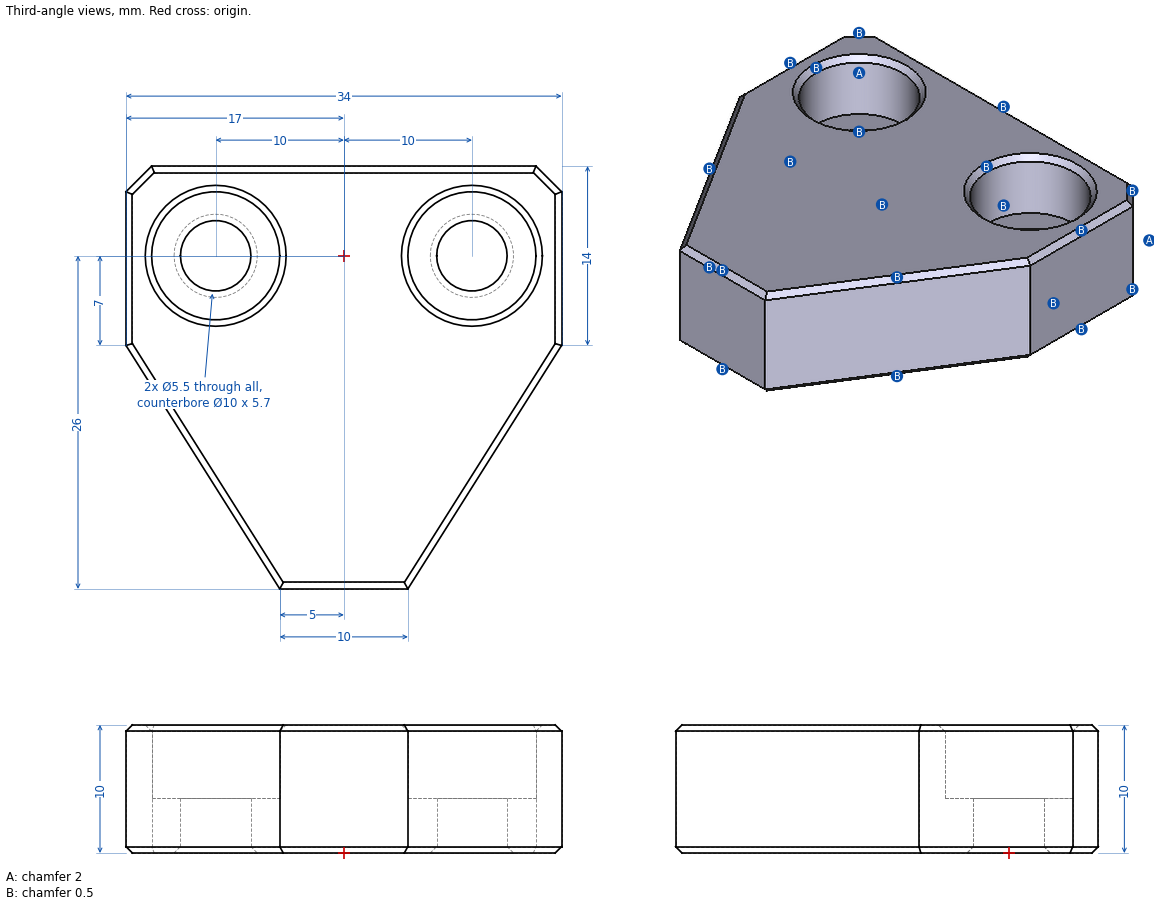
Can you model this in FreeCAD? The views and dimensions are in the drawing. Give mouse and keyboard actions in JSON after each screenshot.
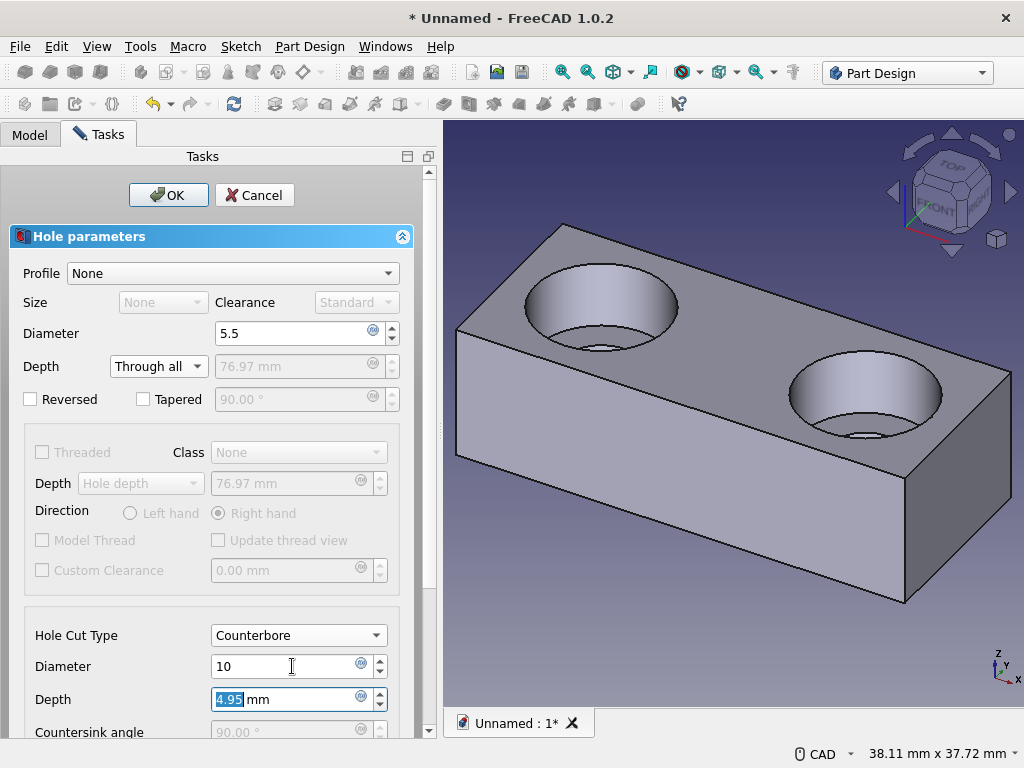
{"action": "type", "text": "5.7"}
{"action": "key", "text": "Tab"}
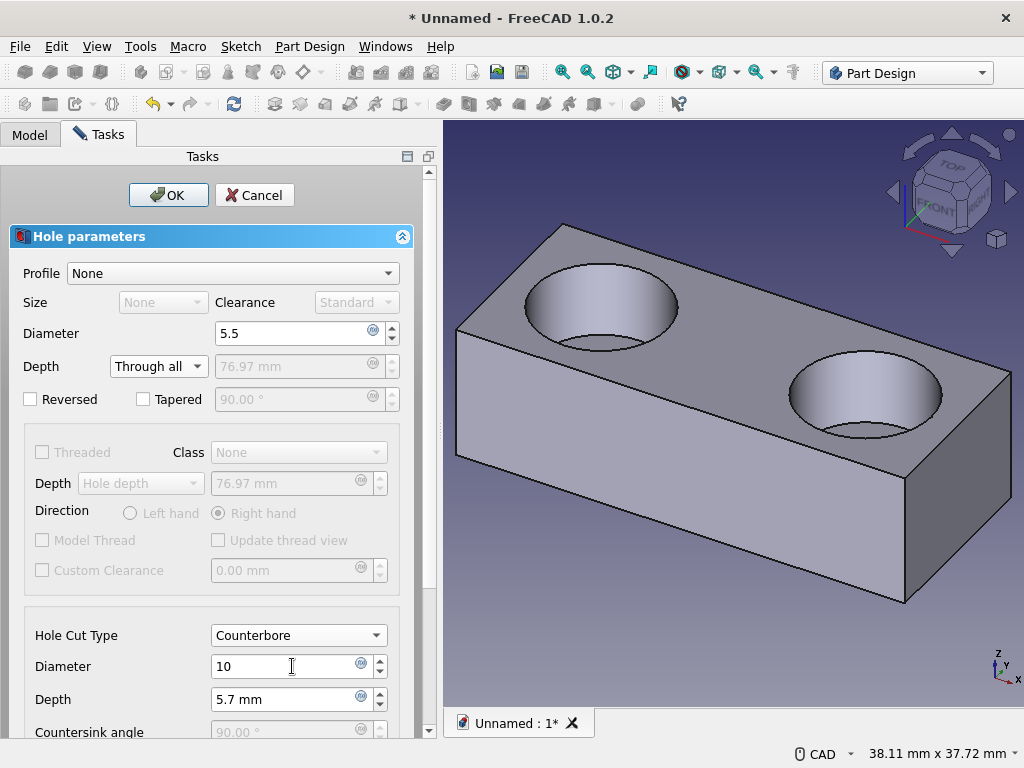
{"action": "left_click", "coordinate": [169, 195]}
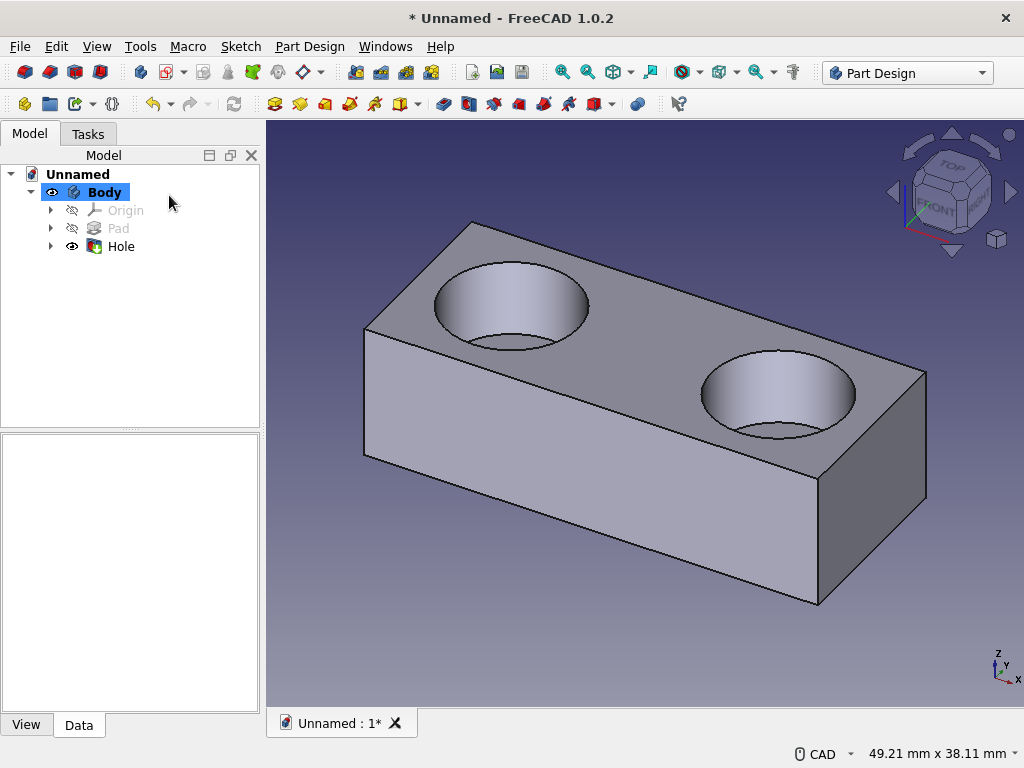
{"action": "left_click", "coordinate": [660, 334]}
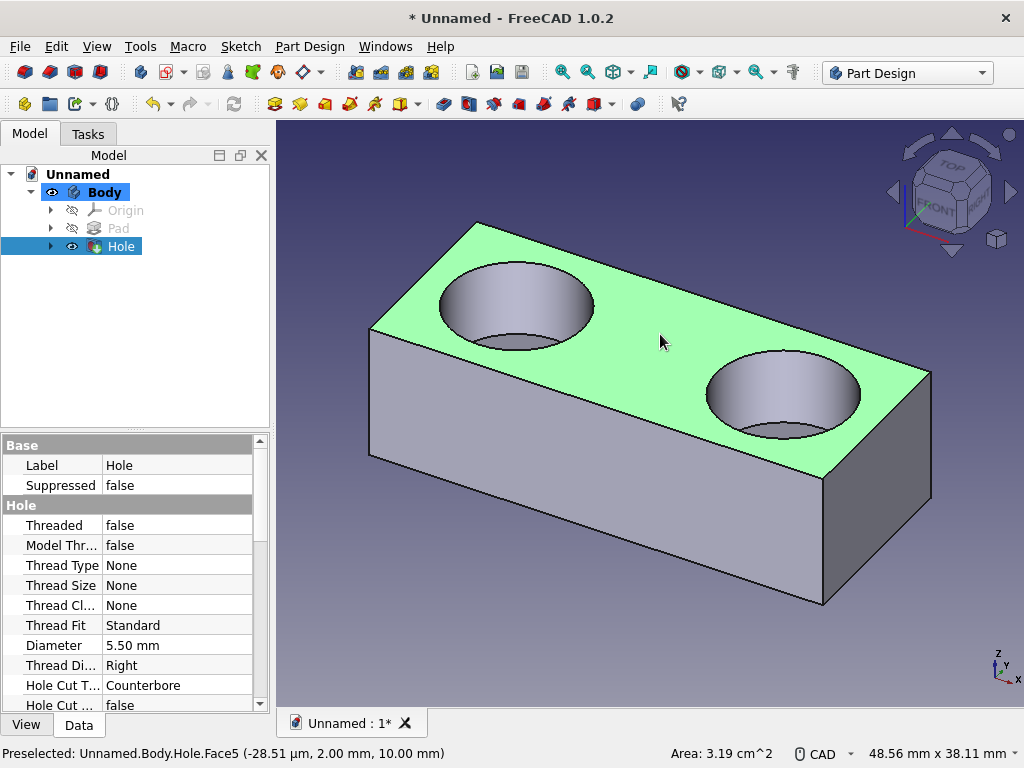
{"action": "left_click", "coordinate": [166, 72]}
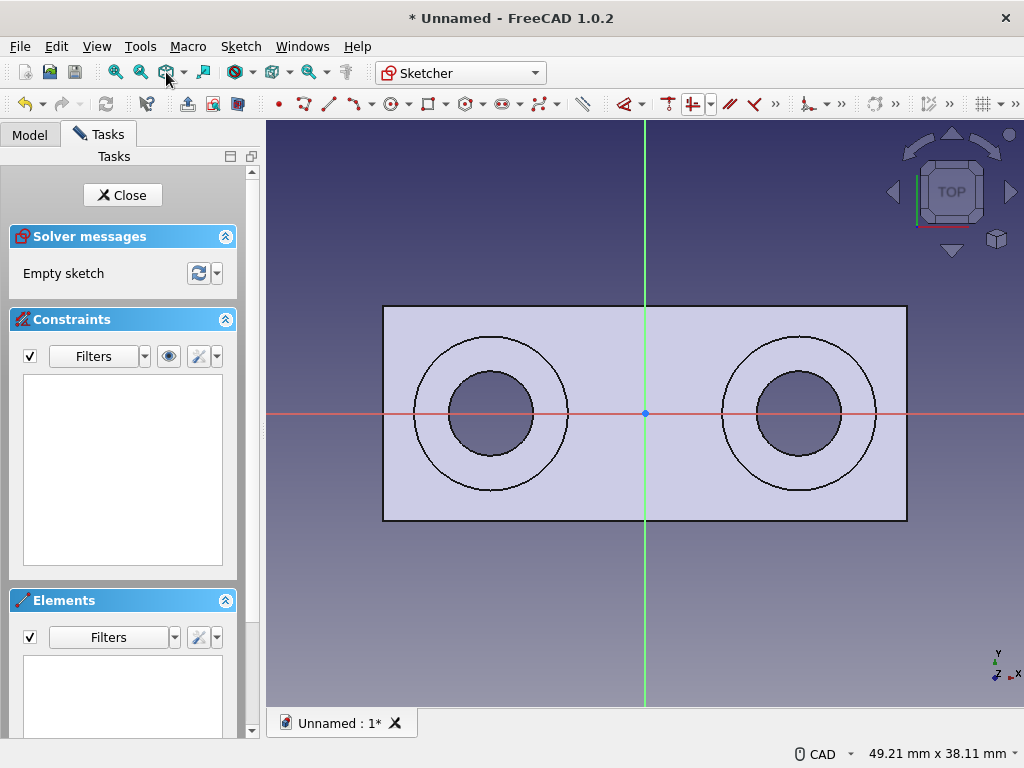
{"action": "scroll", "coordinate": [437, 148], "scroll_direction": "down", "scroll_amount": 2}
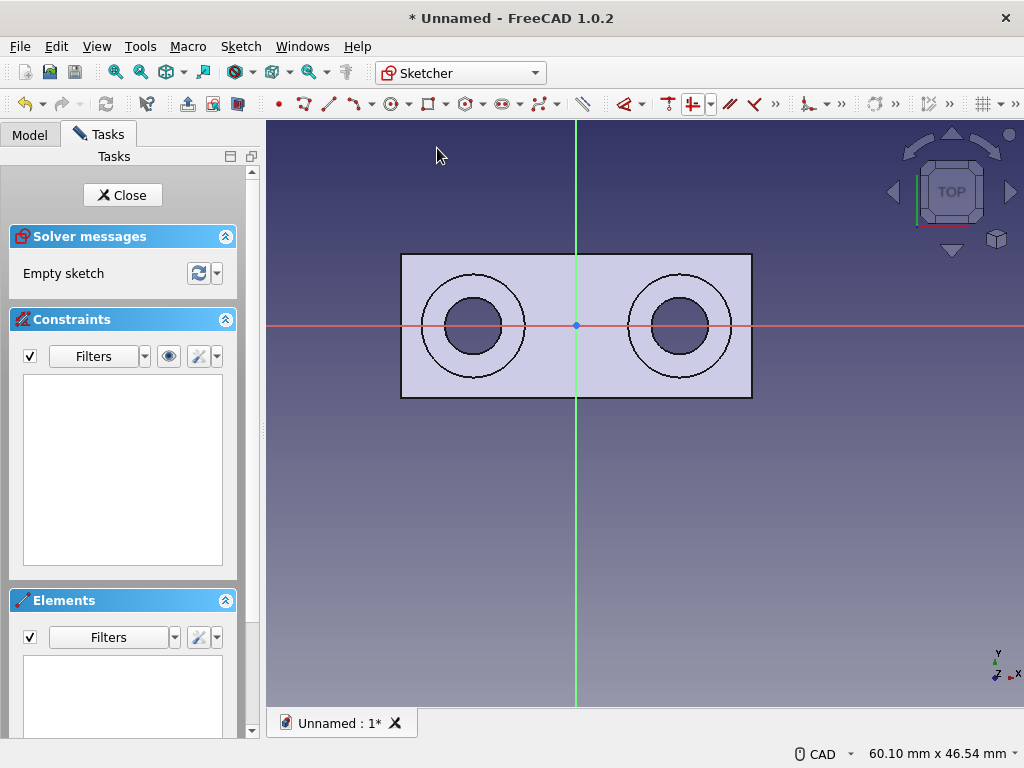
{"action": "left_click", "coordinate": [304, 104]}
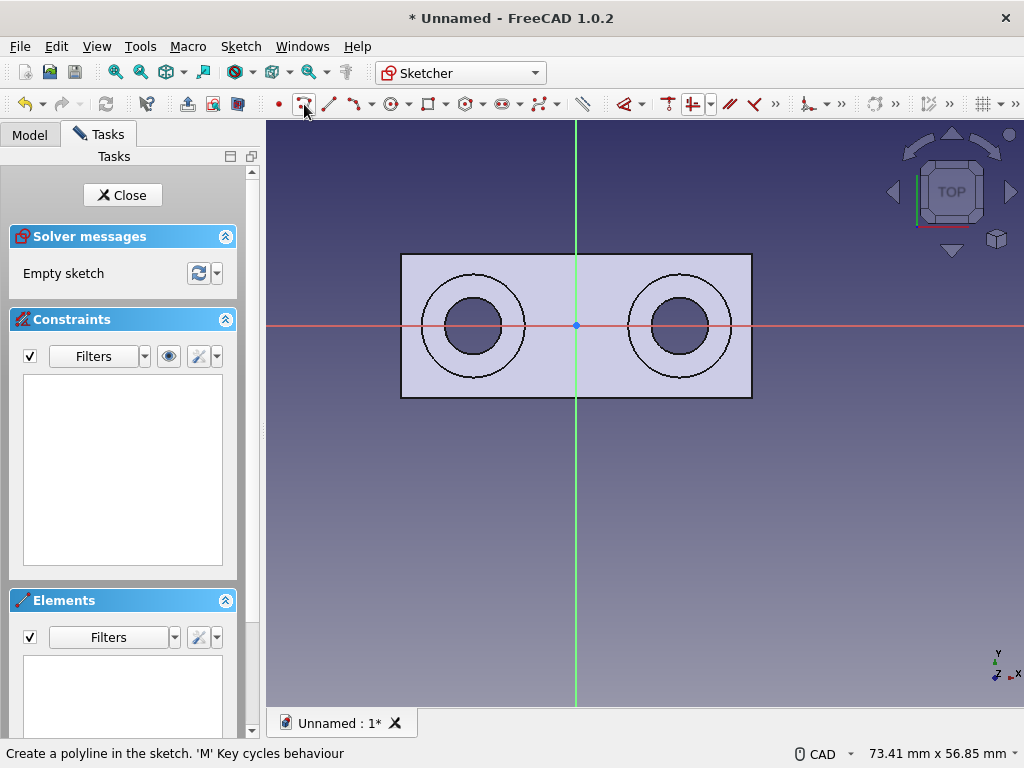
{"action": "left_click", "coordinate": [401, 398]}
{"action": "left_click", "coordinate": [525, 594]}
{"action": "left_click", "coordinate": [628, 594]}
{"action": "left_click", "coordinate": [752, 398]}
{"action": "left_click", "coordinate": [401, 399]}
{"action": "key", "text": "Escape"}
{"action": "key", "text": "Escape"}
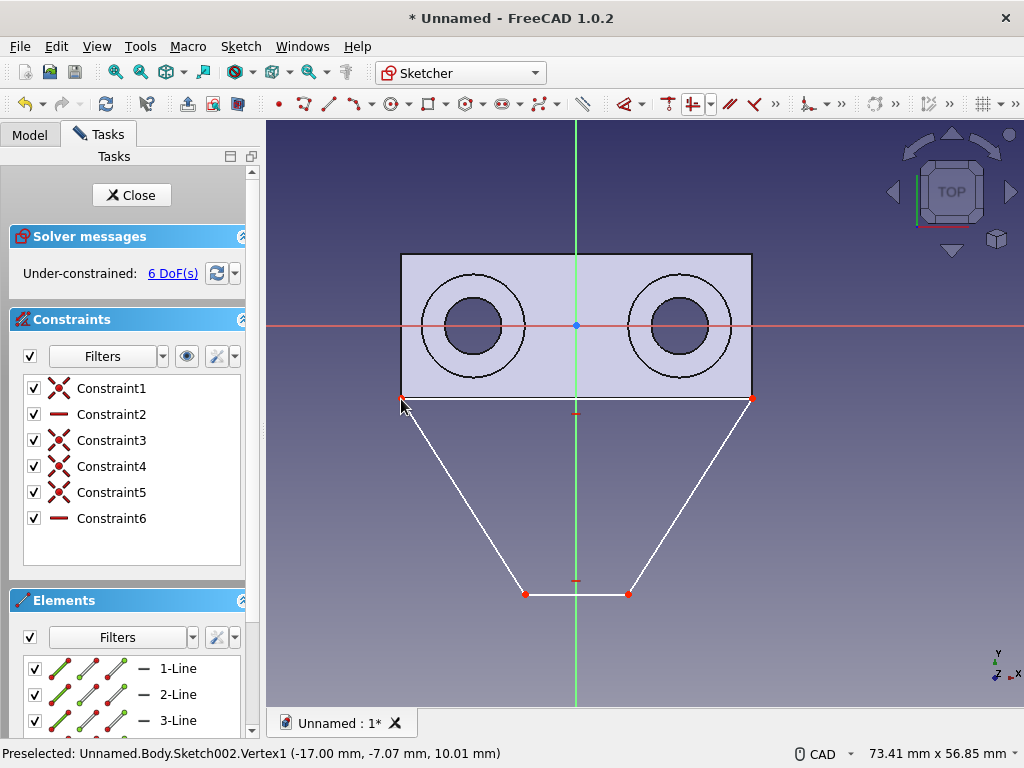
{"action": "left_click", "coordinate": [624, 104]}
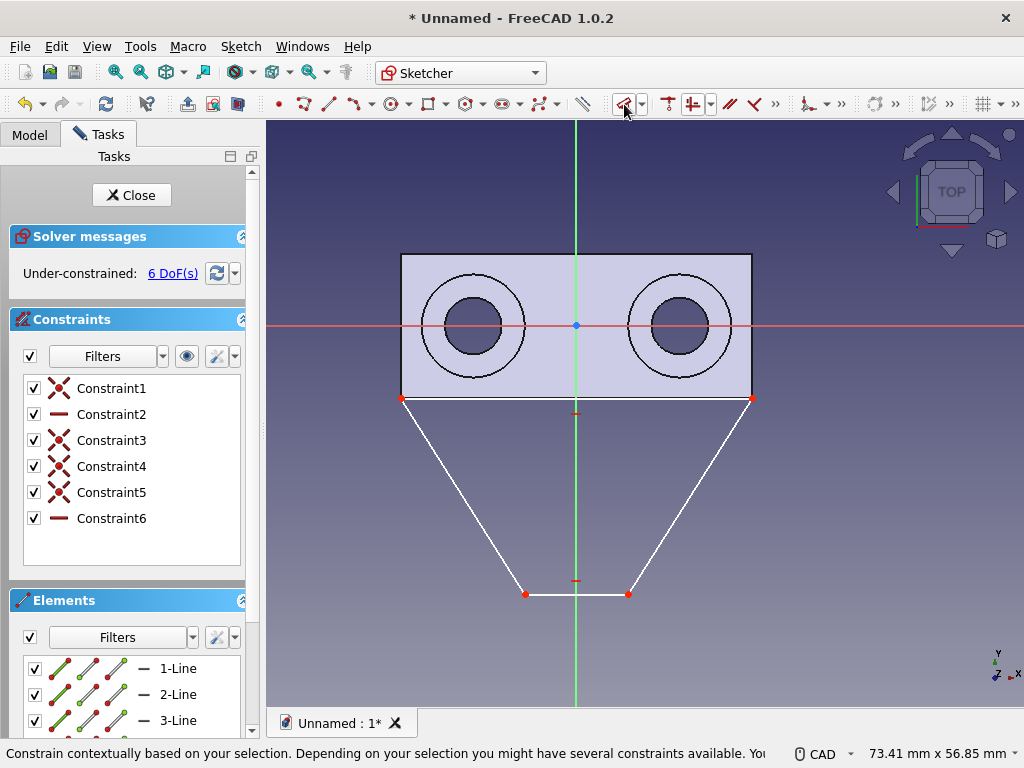
{"action": "left_click", "coordinate": [556, 595]}
{"action": "left_click", "coordinate": [553, 629]}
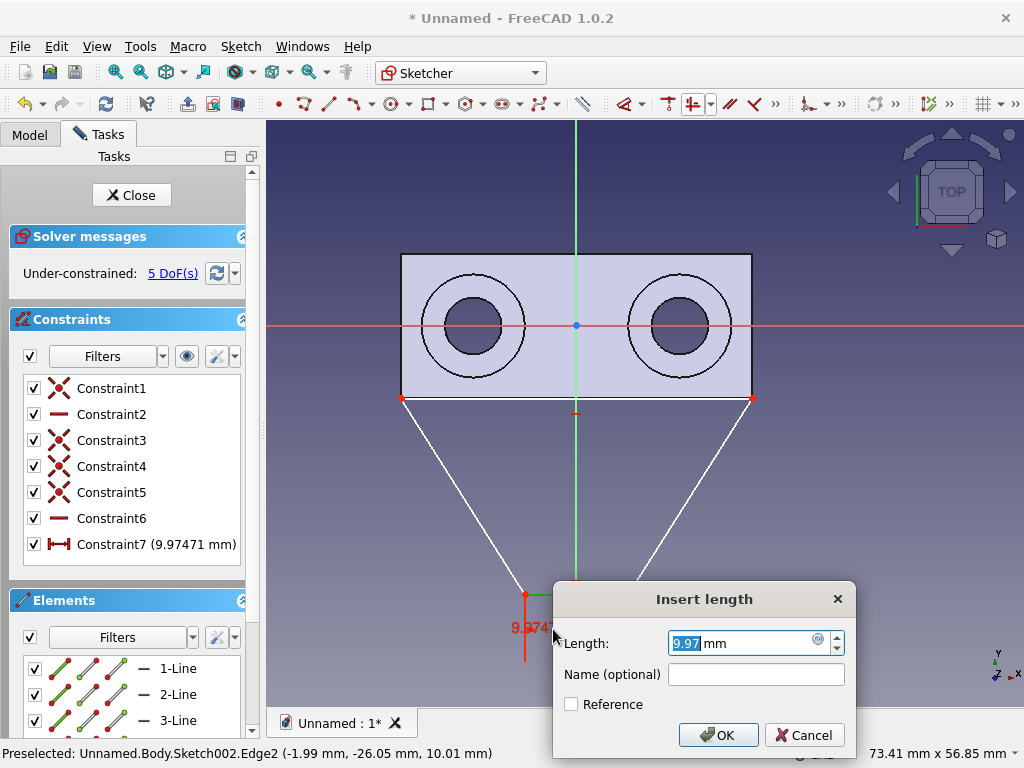
{"action": "type", "text": "10"}
{"action": "key", "text": "Return"}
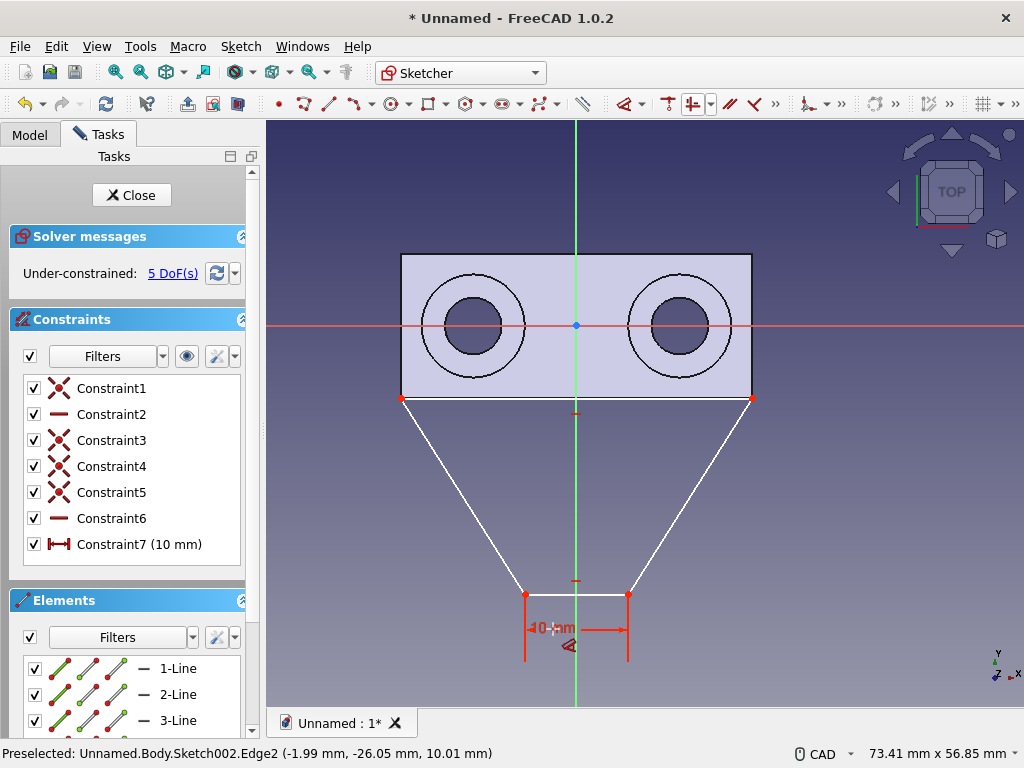
{"action": "left_click", "coordinate": [647, 399]}
{"action": "left_click", "coordinate": [496, 365]}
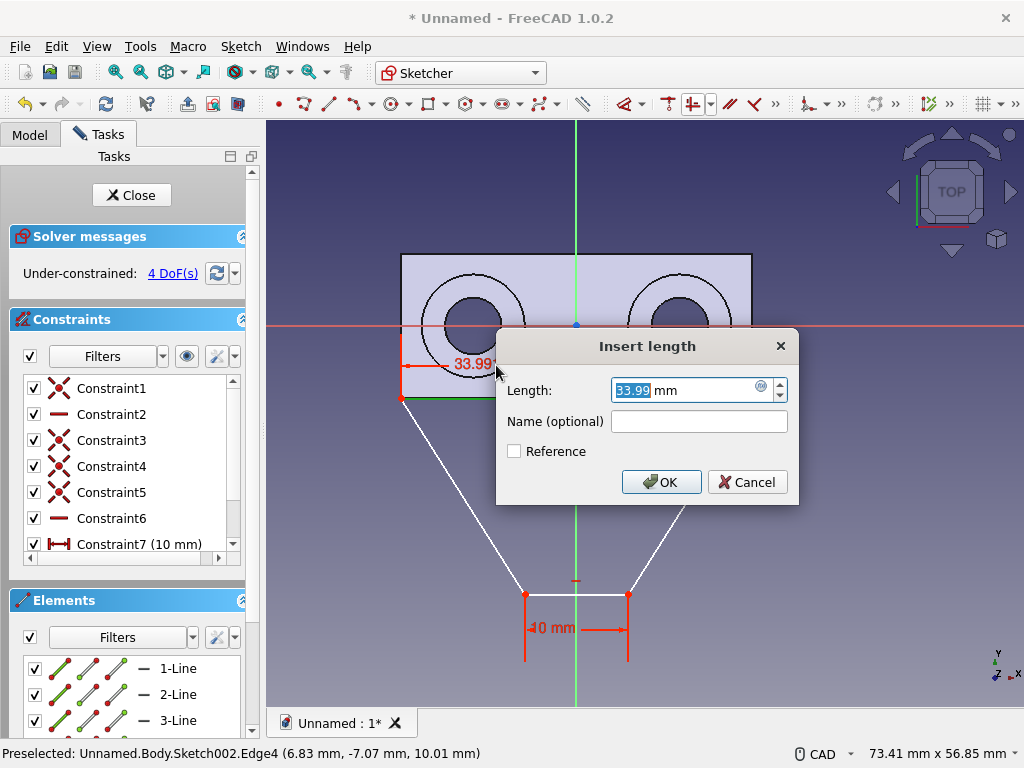
{"action": "type", "text": "34"}
{"action": "key", "text": "Return"}